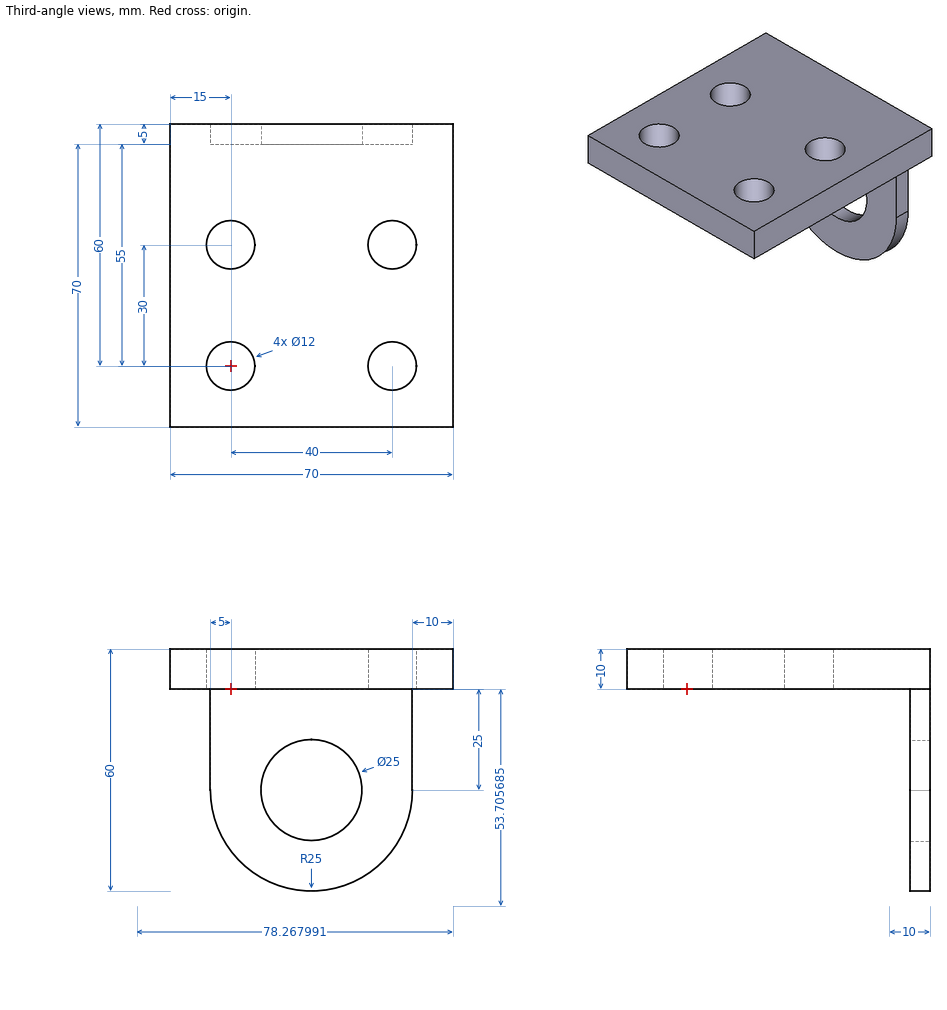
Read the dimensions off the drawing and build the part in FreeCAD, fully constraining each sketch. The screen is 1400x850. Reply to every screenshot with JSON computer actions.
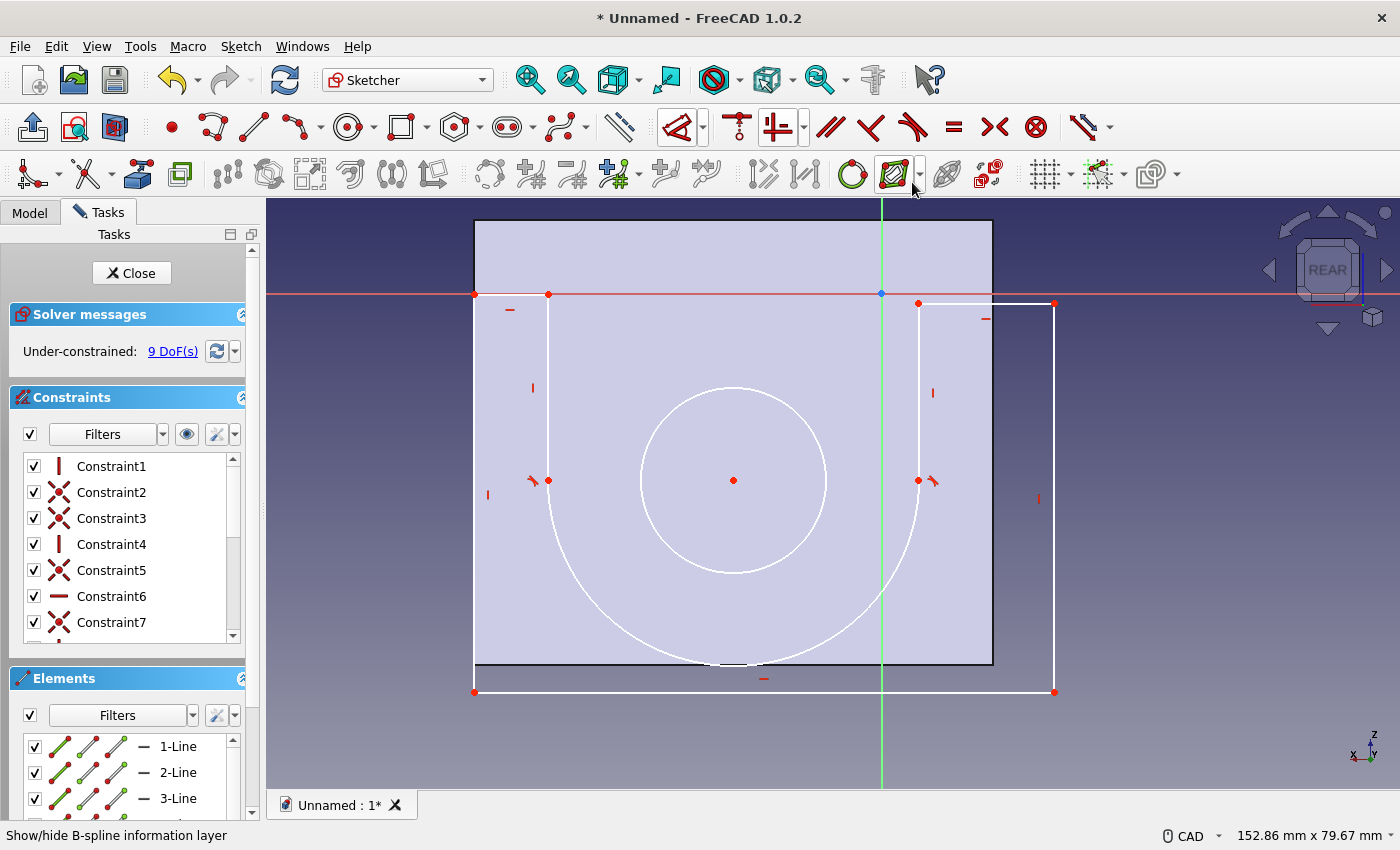
{"action": "left_click", "coordinate": [624, 631]}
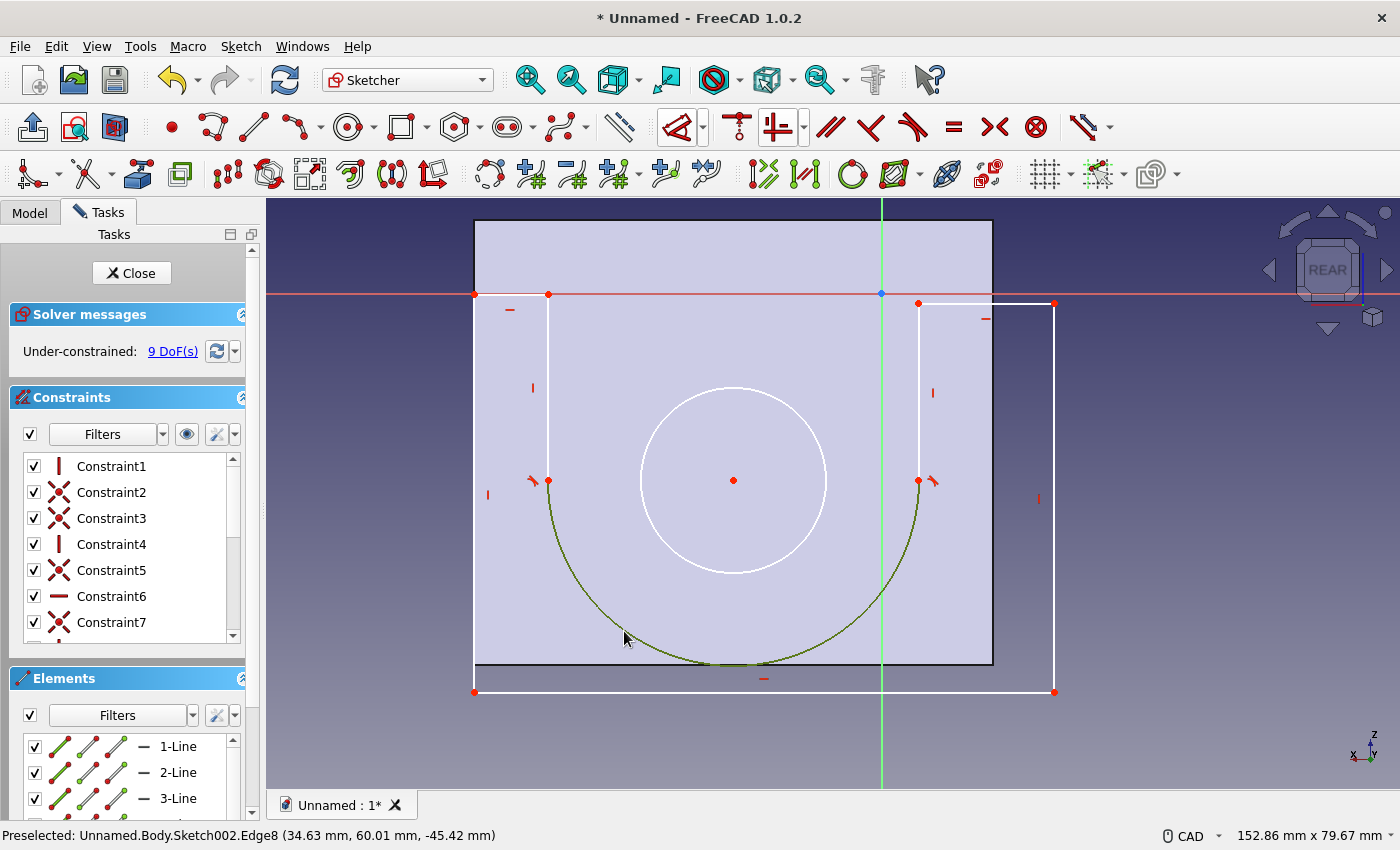
{"action": "left_click", "coordinate": [702, 128]}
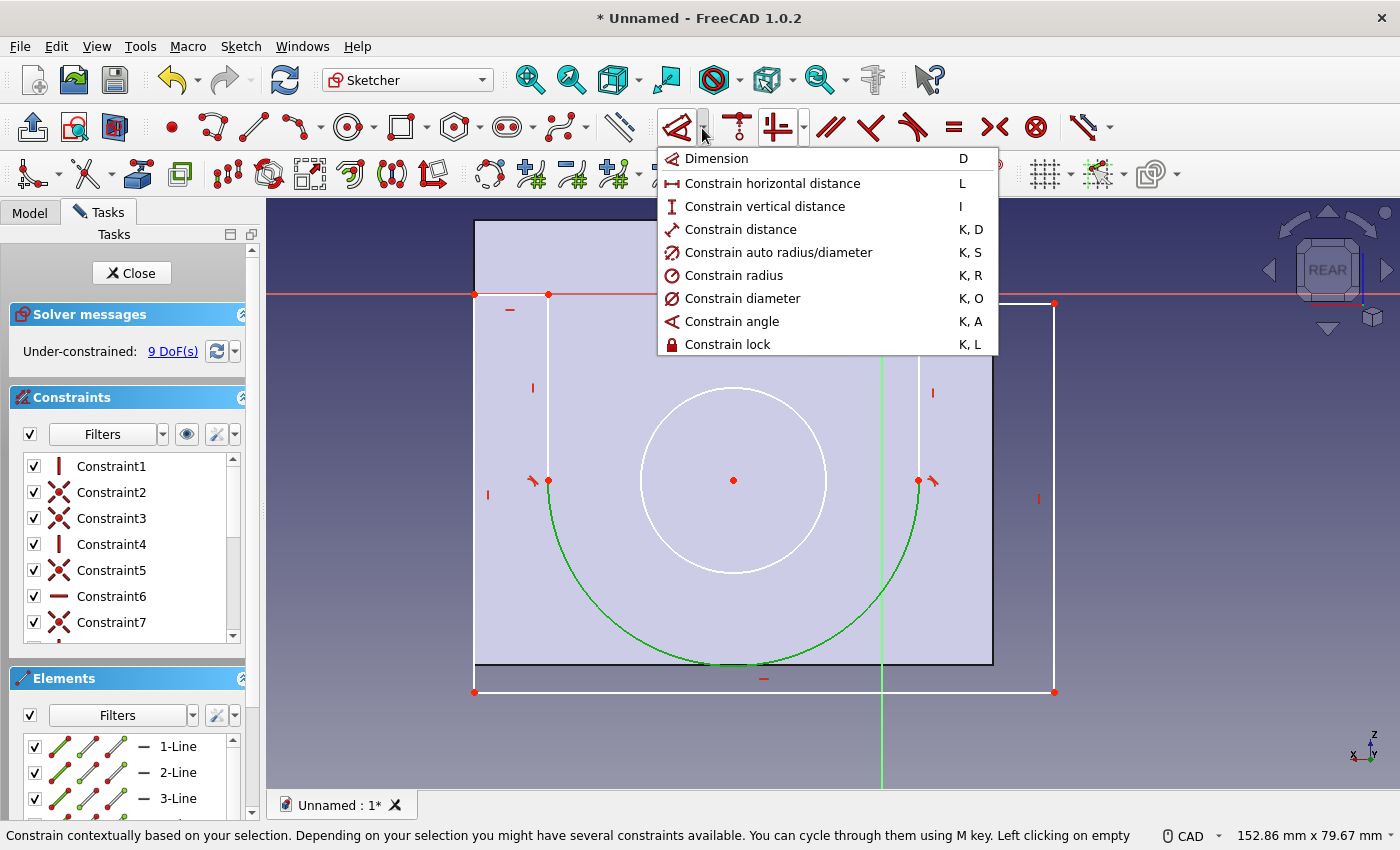
{"action": "left_click", "coordinate": [828, 276]}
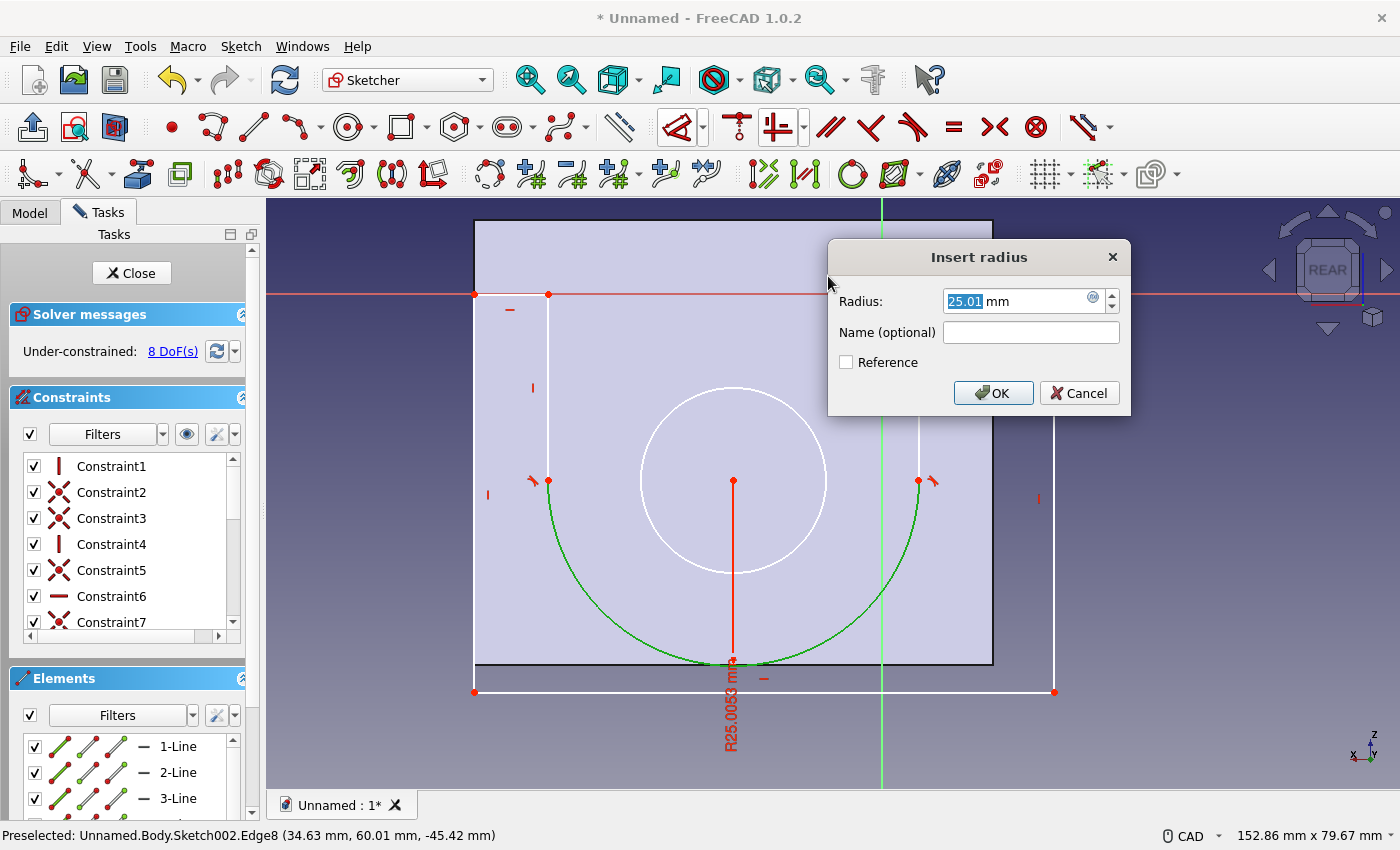
{"action": "type", "text": "25"}
{"action": "key", "text": "Return"}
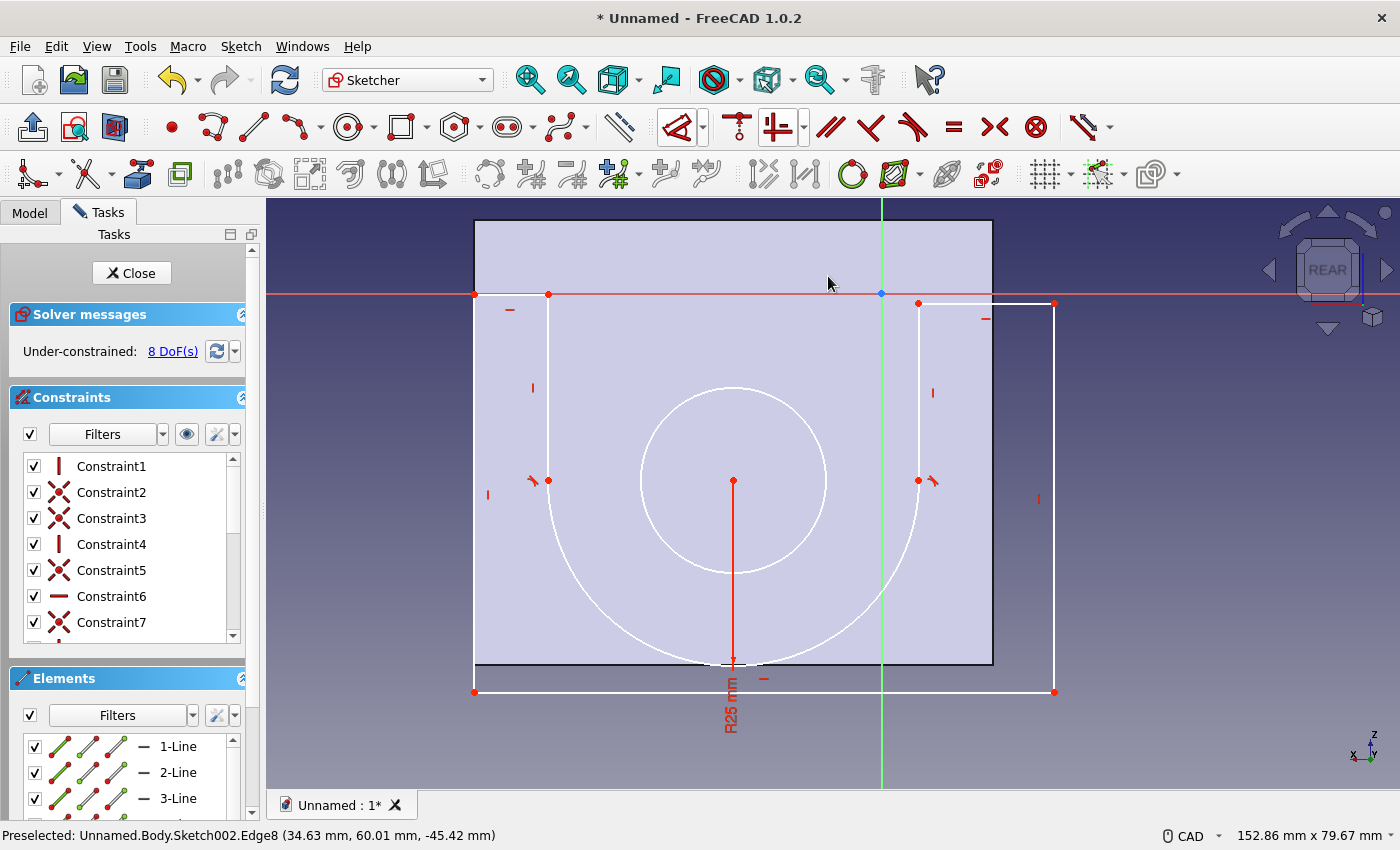
{"action": "left_click", "coordinate": [799, 415]}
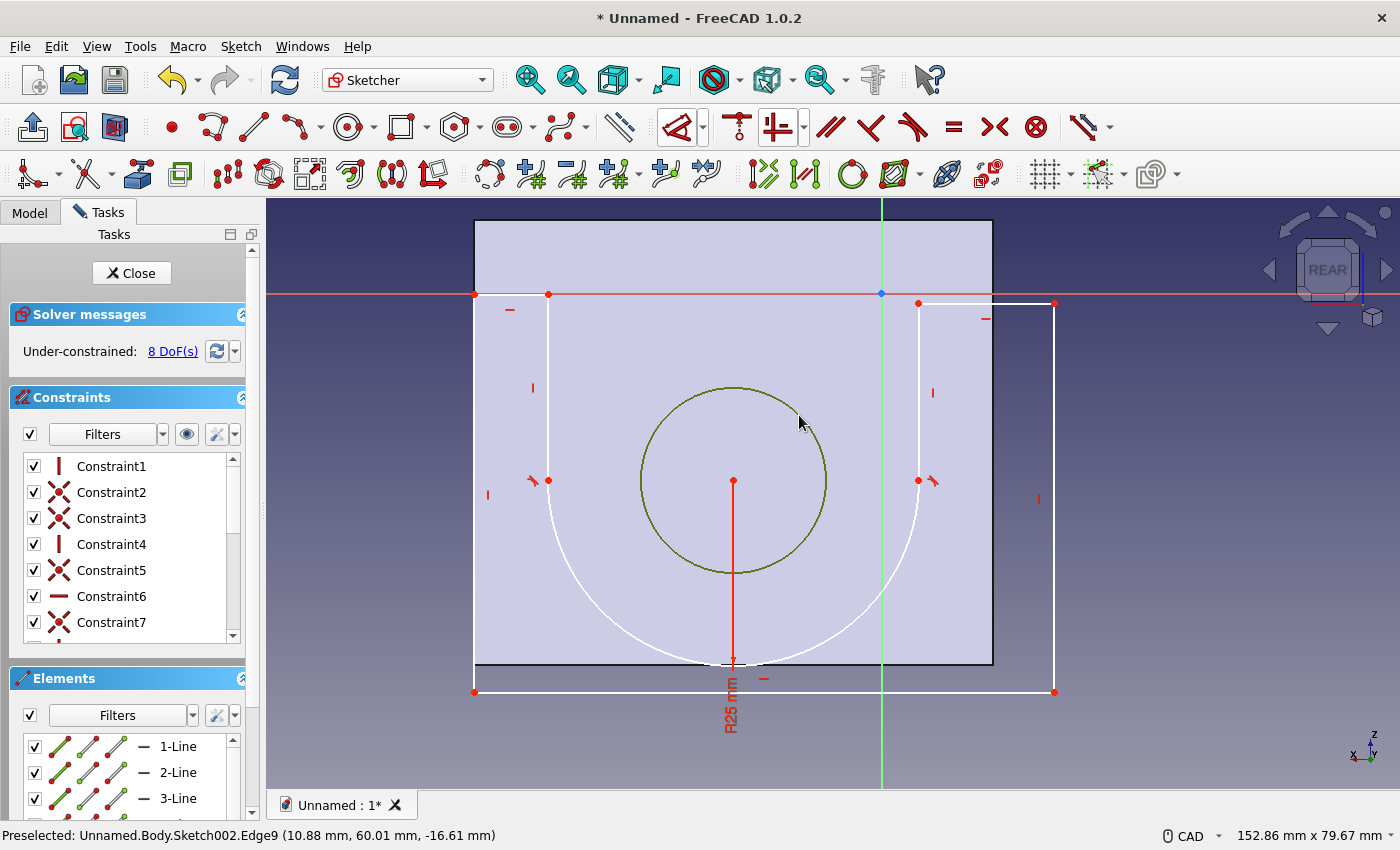
{"action": "key", "text": "k o"}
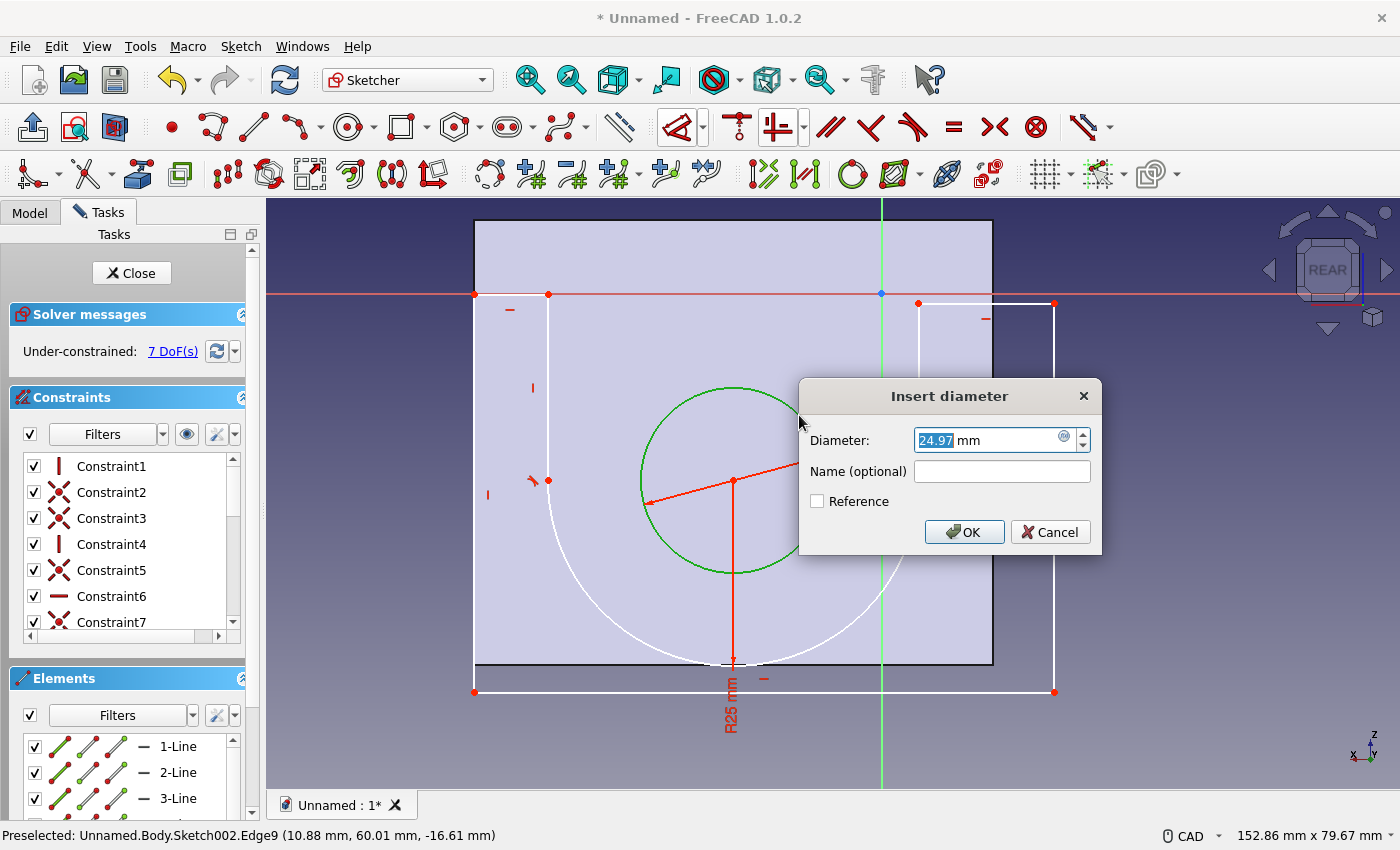
{"action": "type", "text": "25"}
{"action": "key", "text": "Return"}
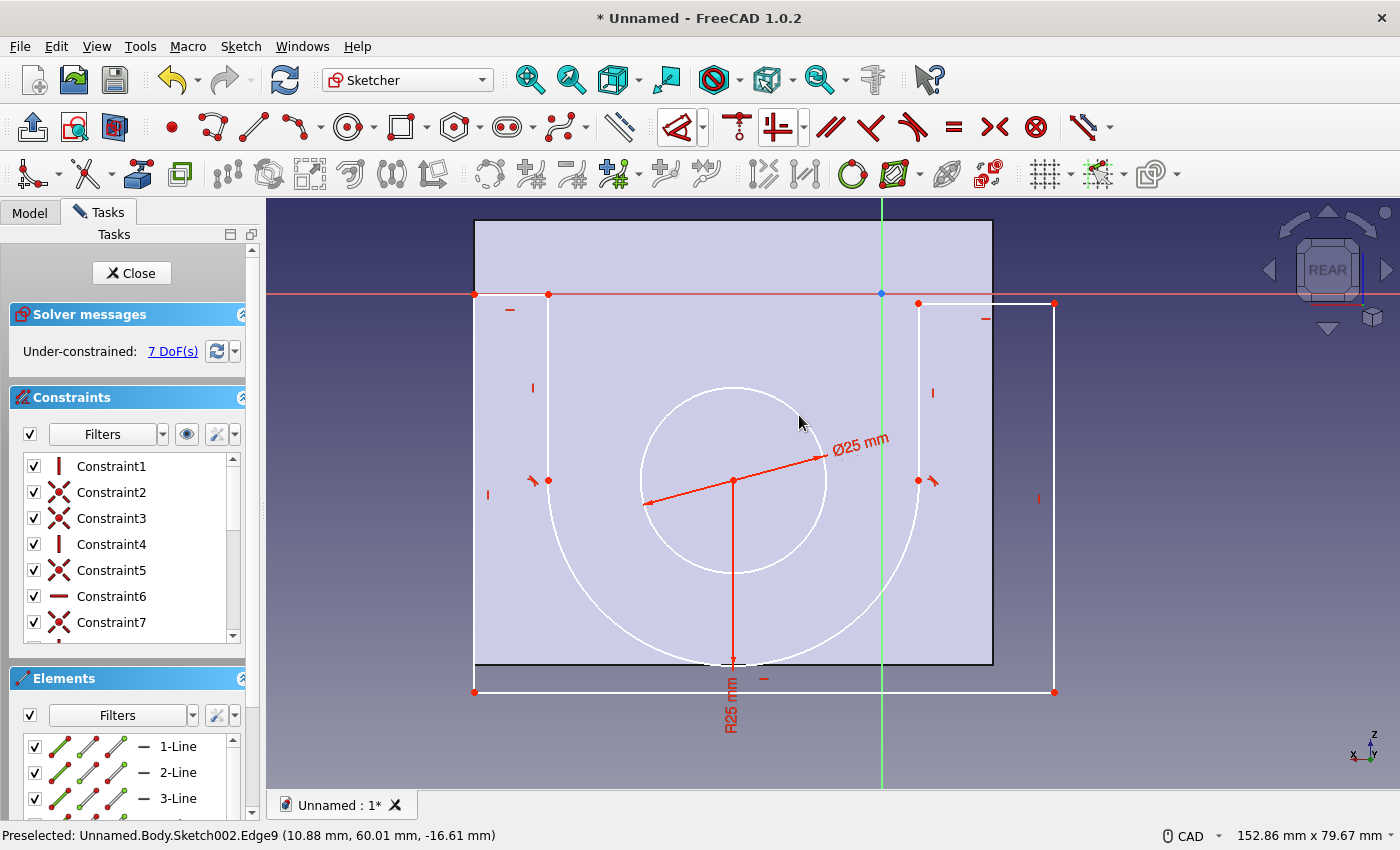
{"action": "left_click", "coordinate": [548, 295]}